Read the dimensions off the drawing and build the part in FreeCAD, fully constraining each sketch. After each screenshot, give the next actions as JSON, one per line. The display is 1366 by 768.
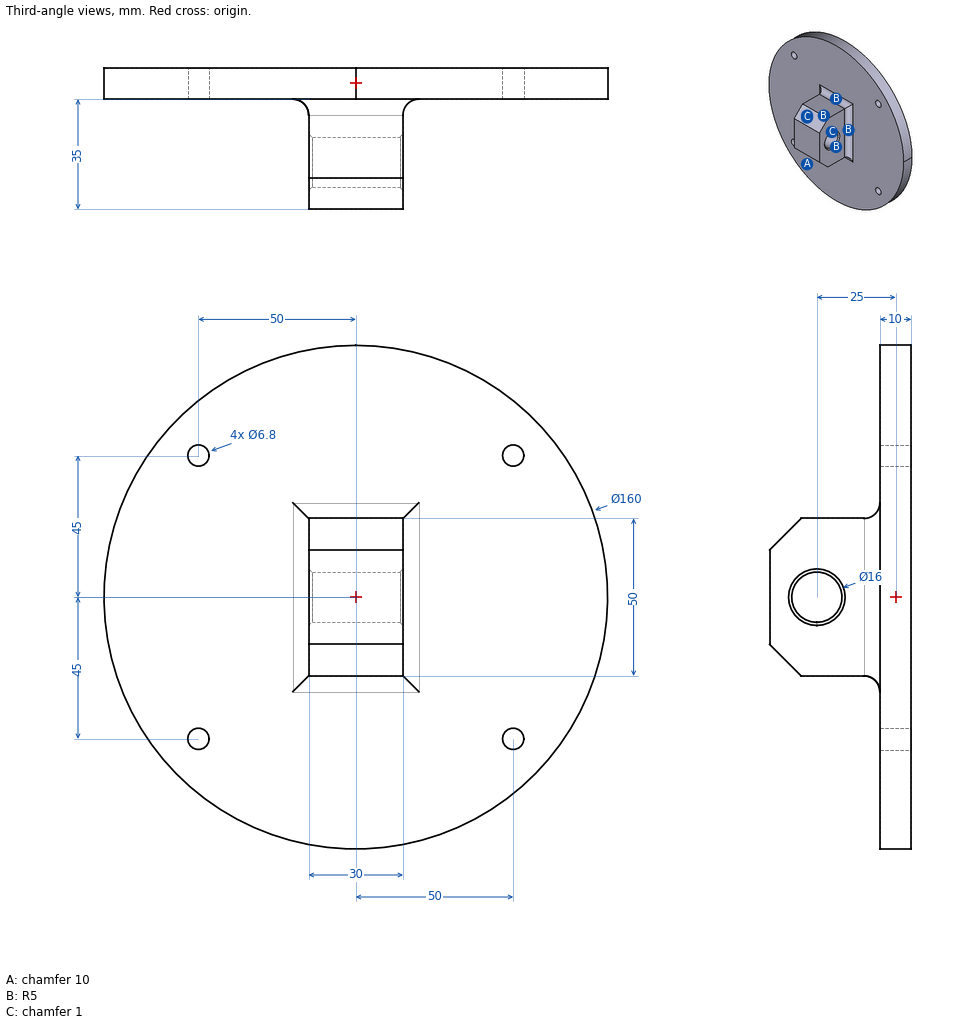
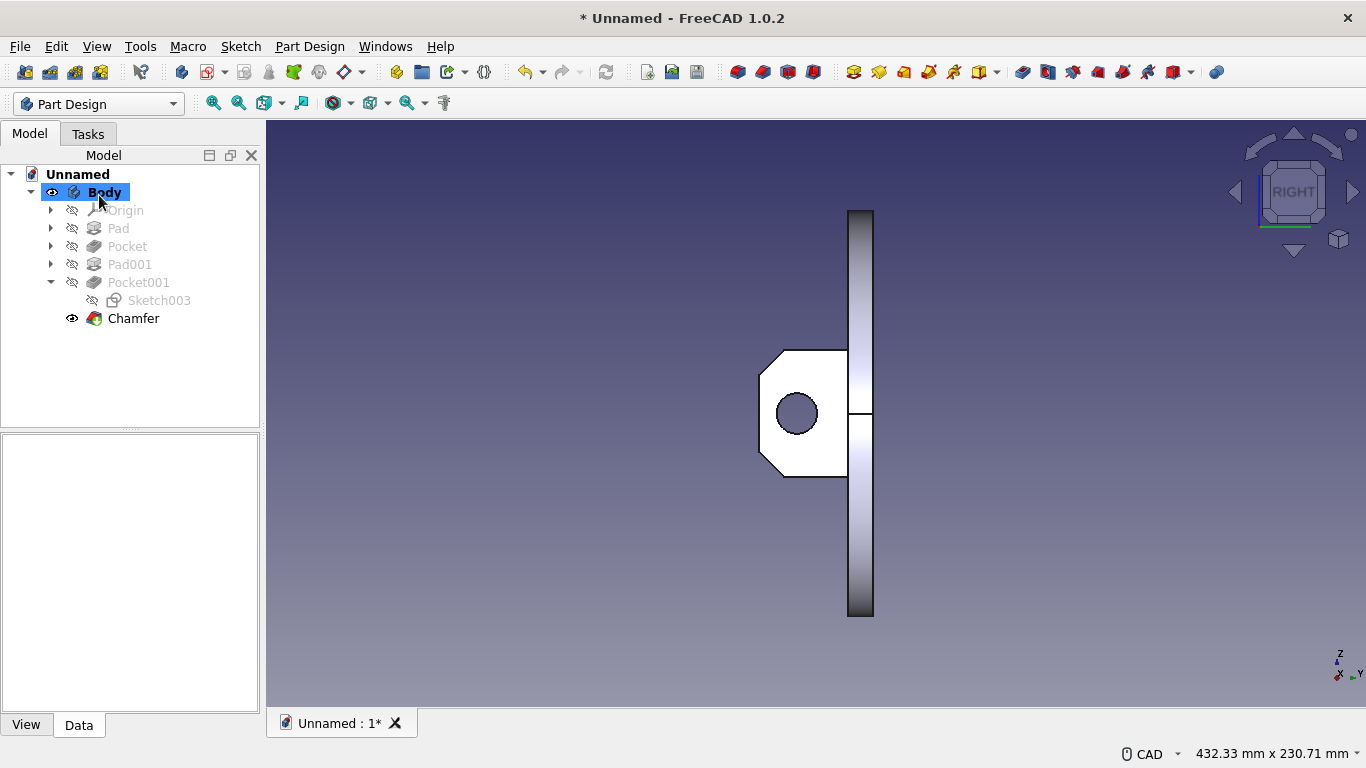
{"action": "key", "text": "5"}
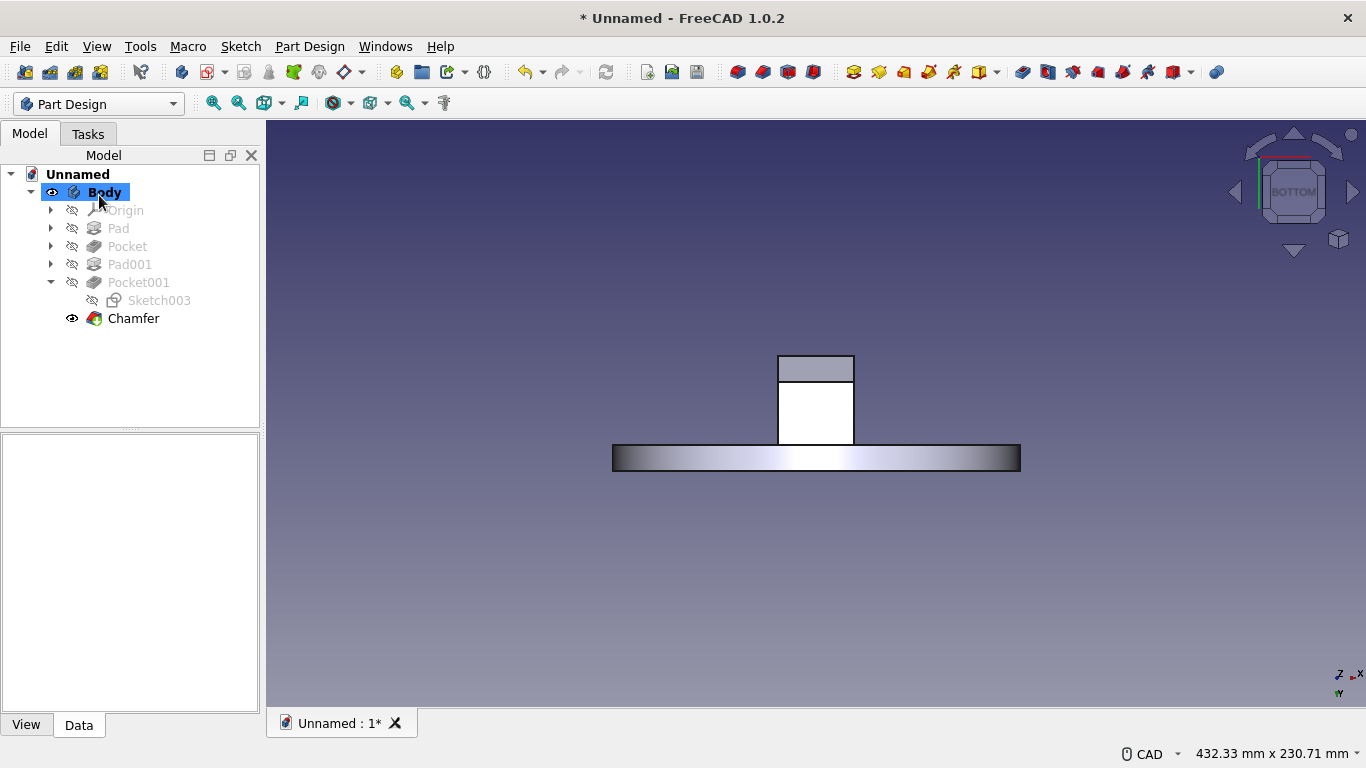
{"action": "left_click", "coordinate": [214, 104]}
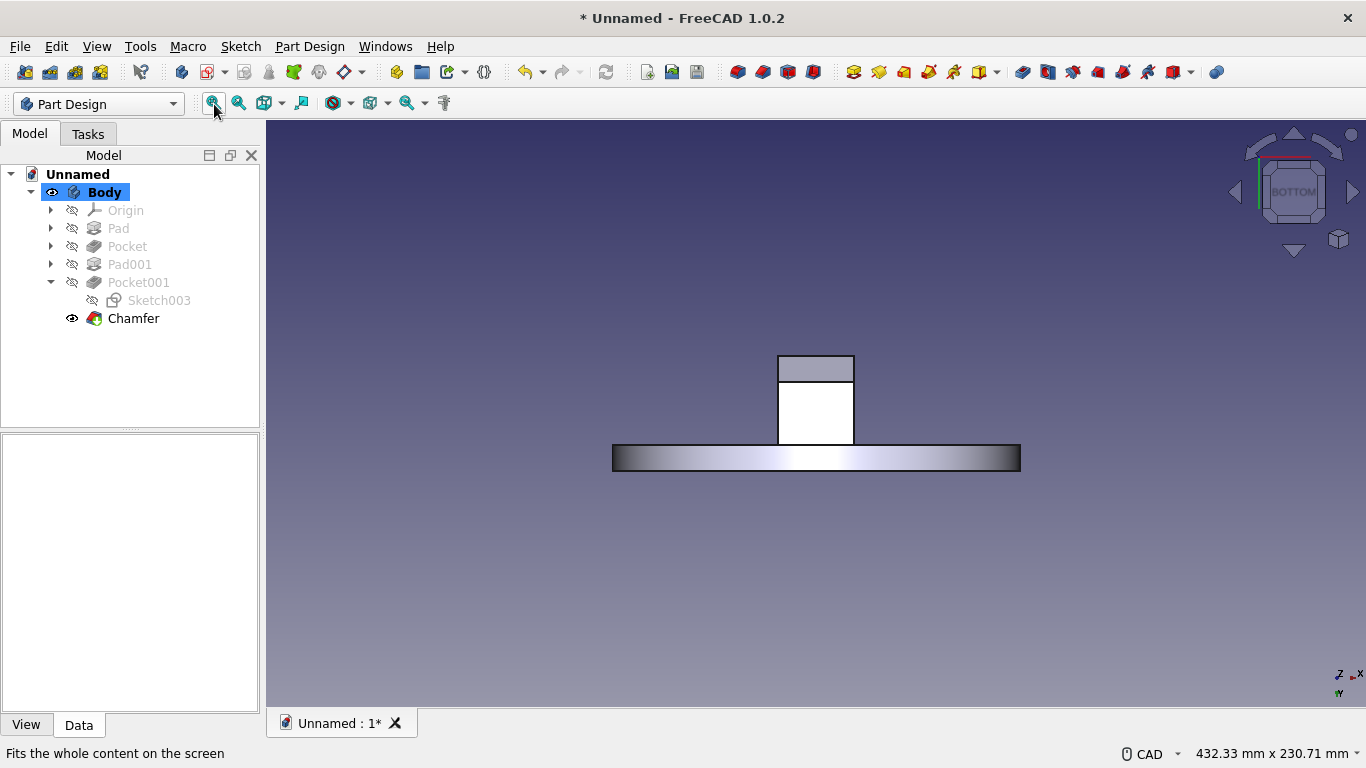
{"action": "key", "text": "4"}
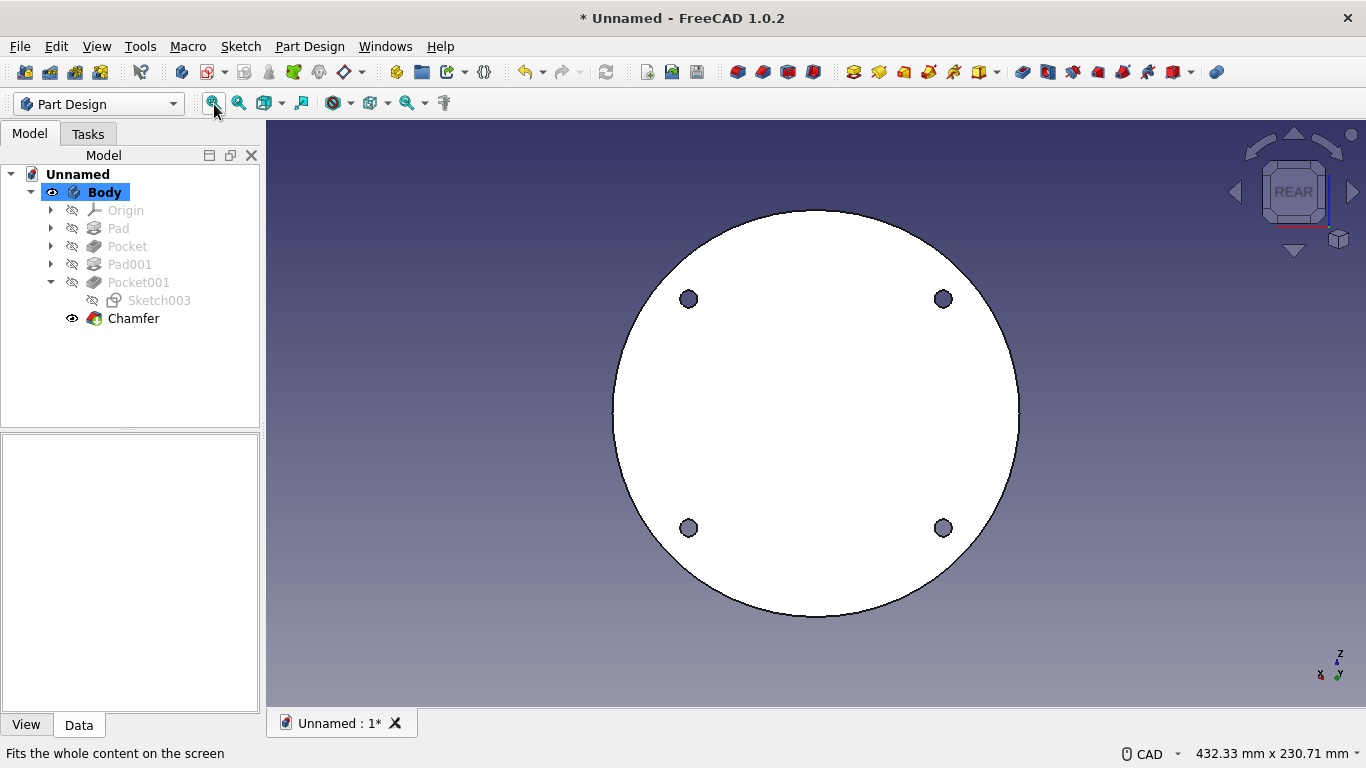
{"action": "key", "text": "6"}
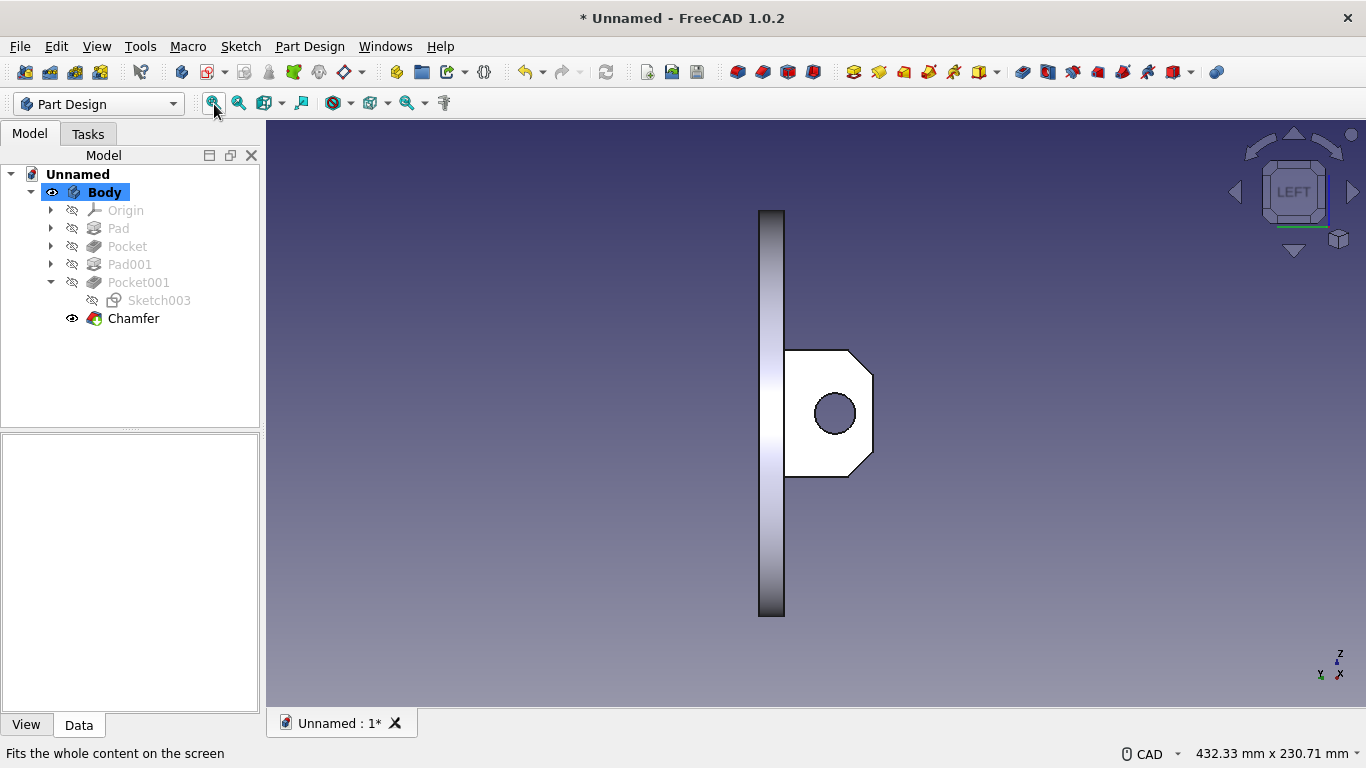
{"action": "key", "text": "v 3"}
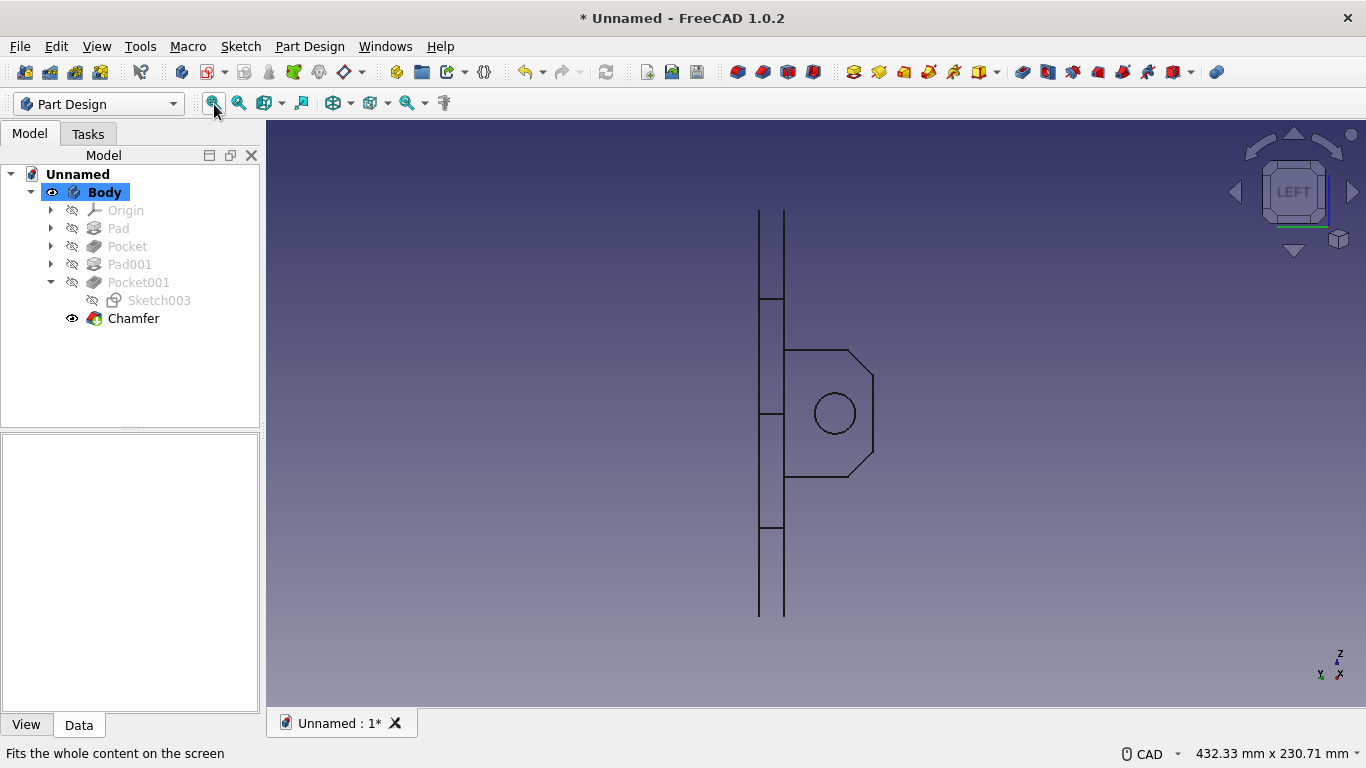
{"action": "key", "text": "0"}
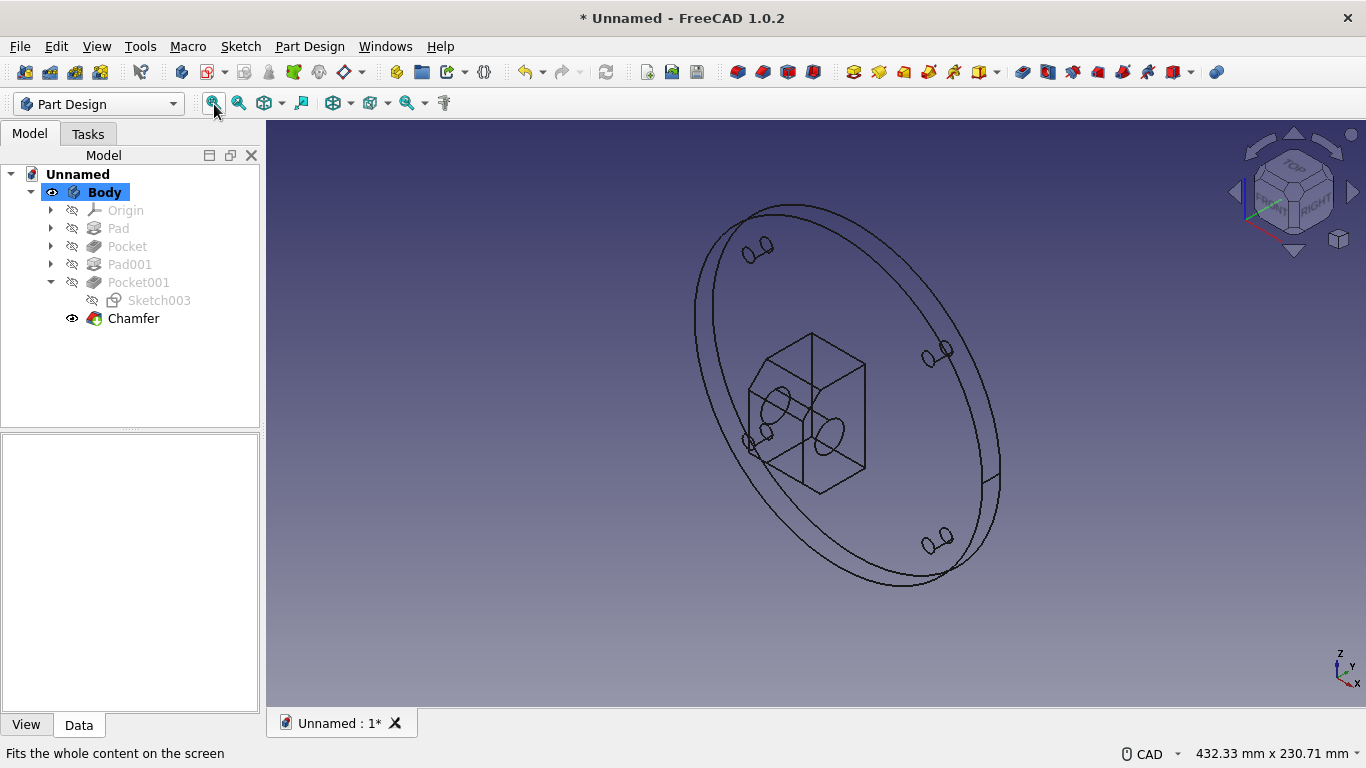
{"action": "left_click", "coordinate": [865, 415]}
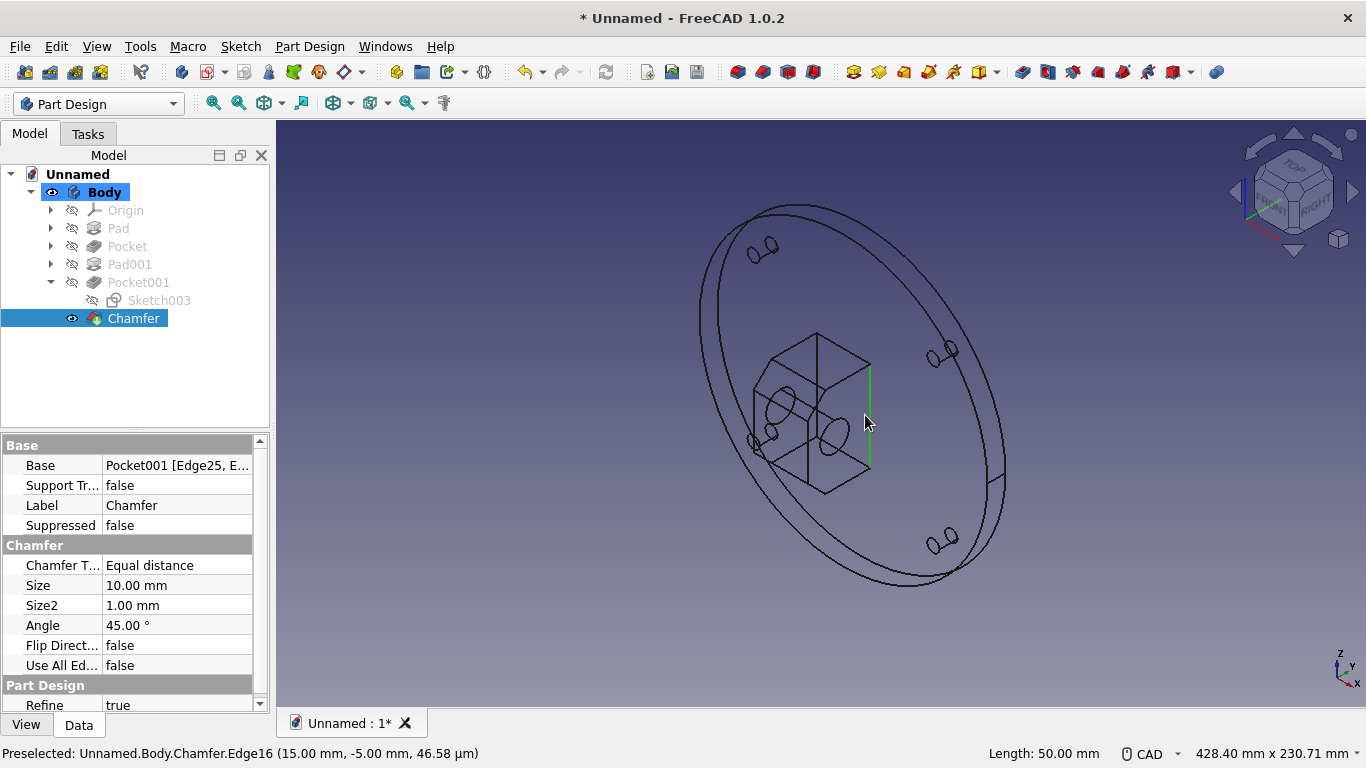
{"action": "left_click", "coordinate": [843, 348], "text": "ctrl"}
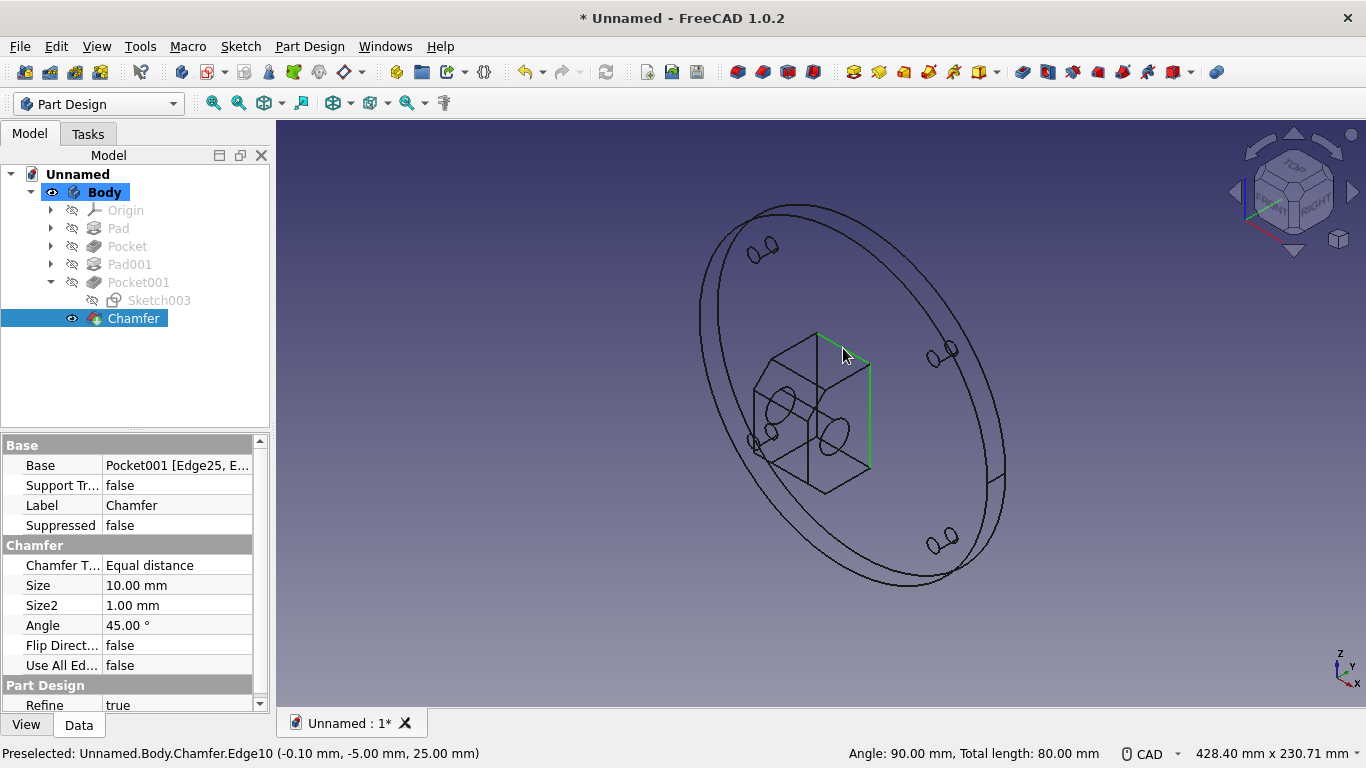
{"action": "left_click", "coordinate": [817, 374], "text": "ctrl"}